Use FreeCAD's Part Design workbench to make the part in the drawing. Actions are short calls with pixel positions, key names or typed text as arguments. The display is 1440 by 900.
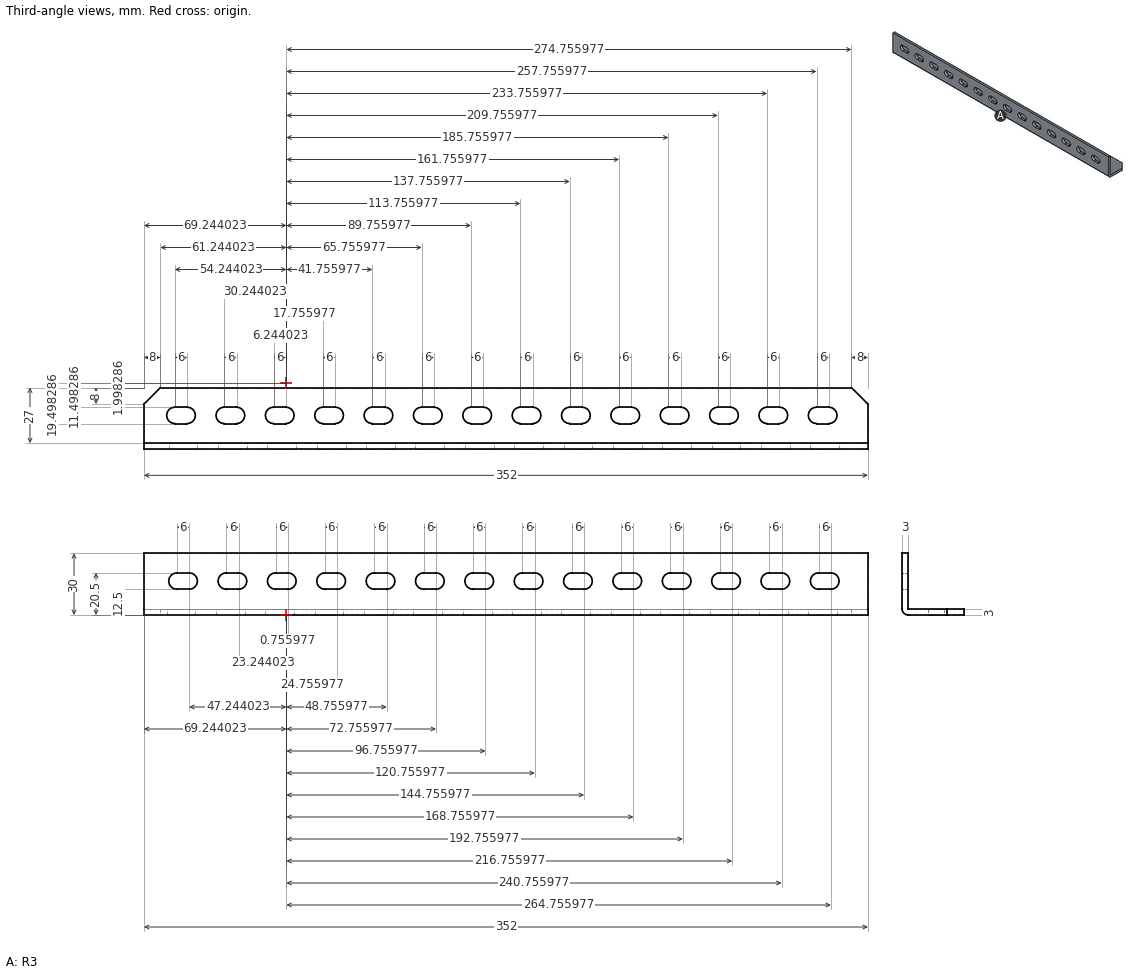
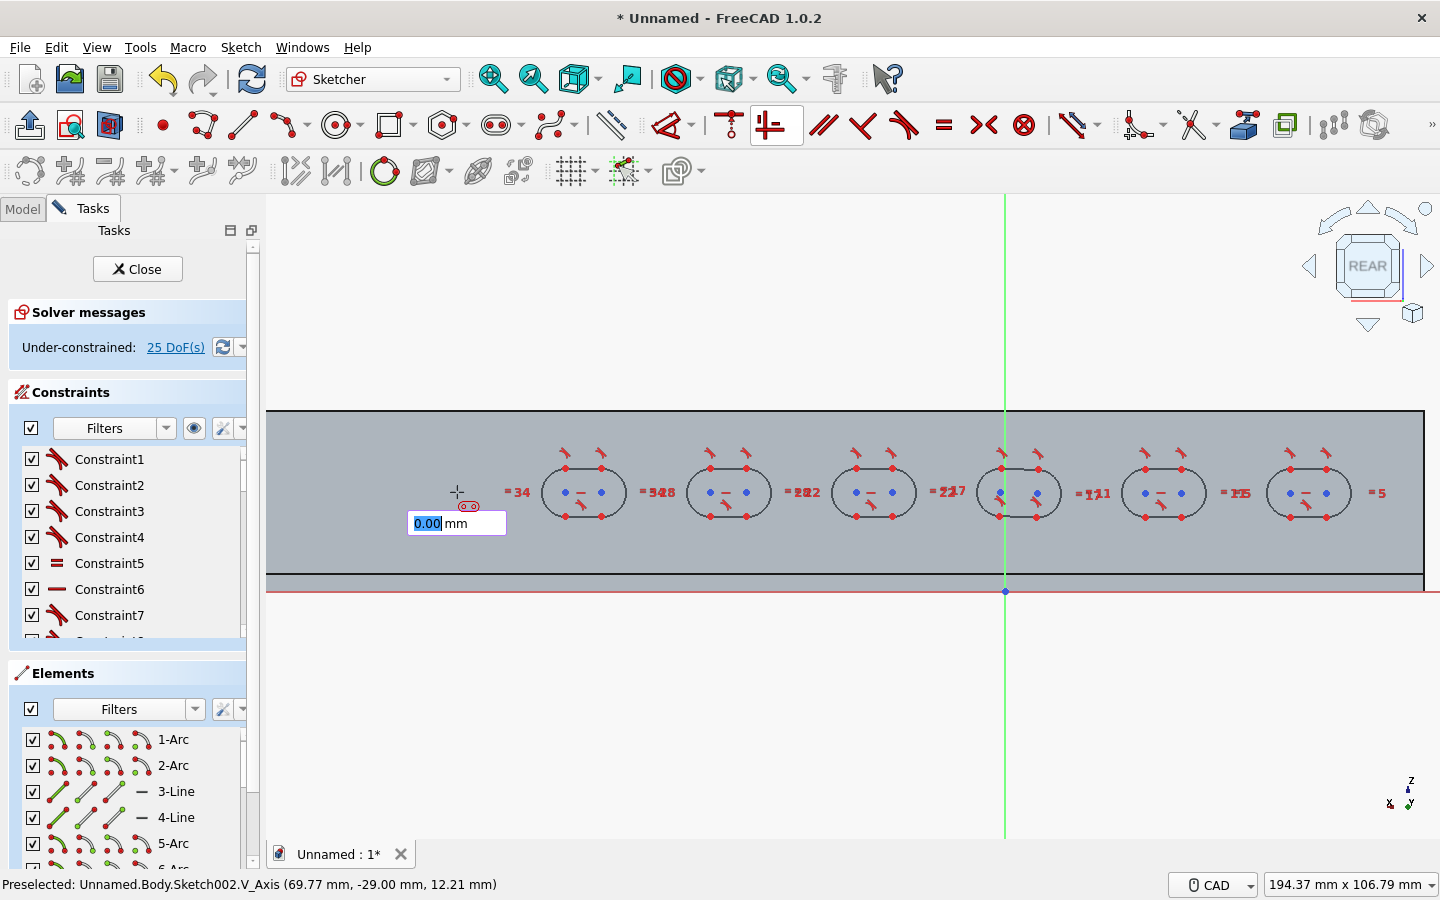
click(439, 516)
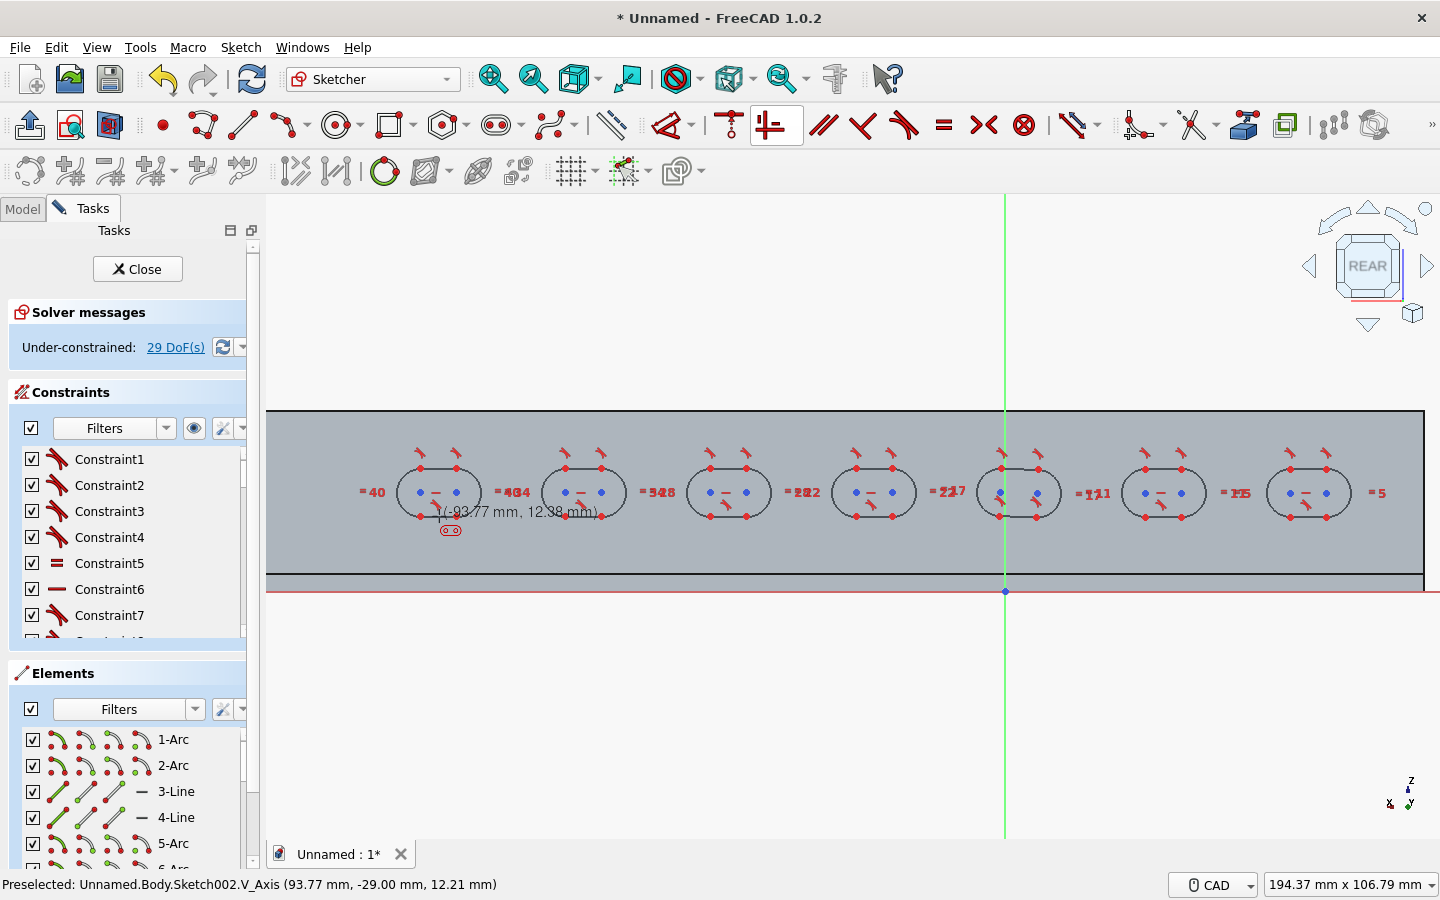
scroll(1028, 509, down, 5)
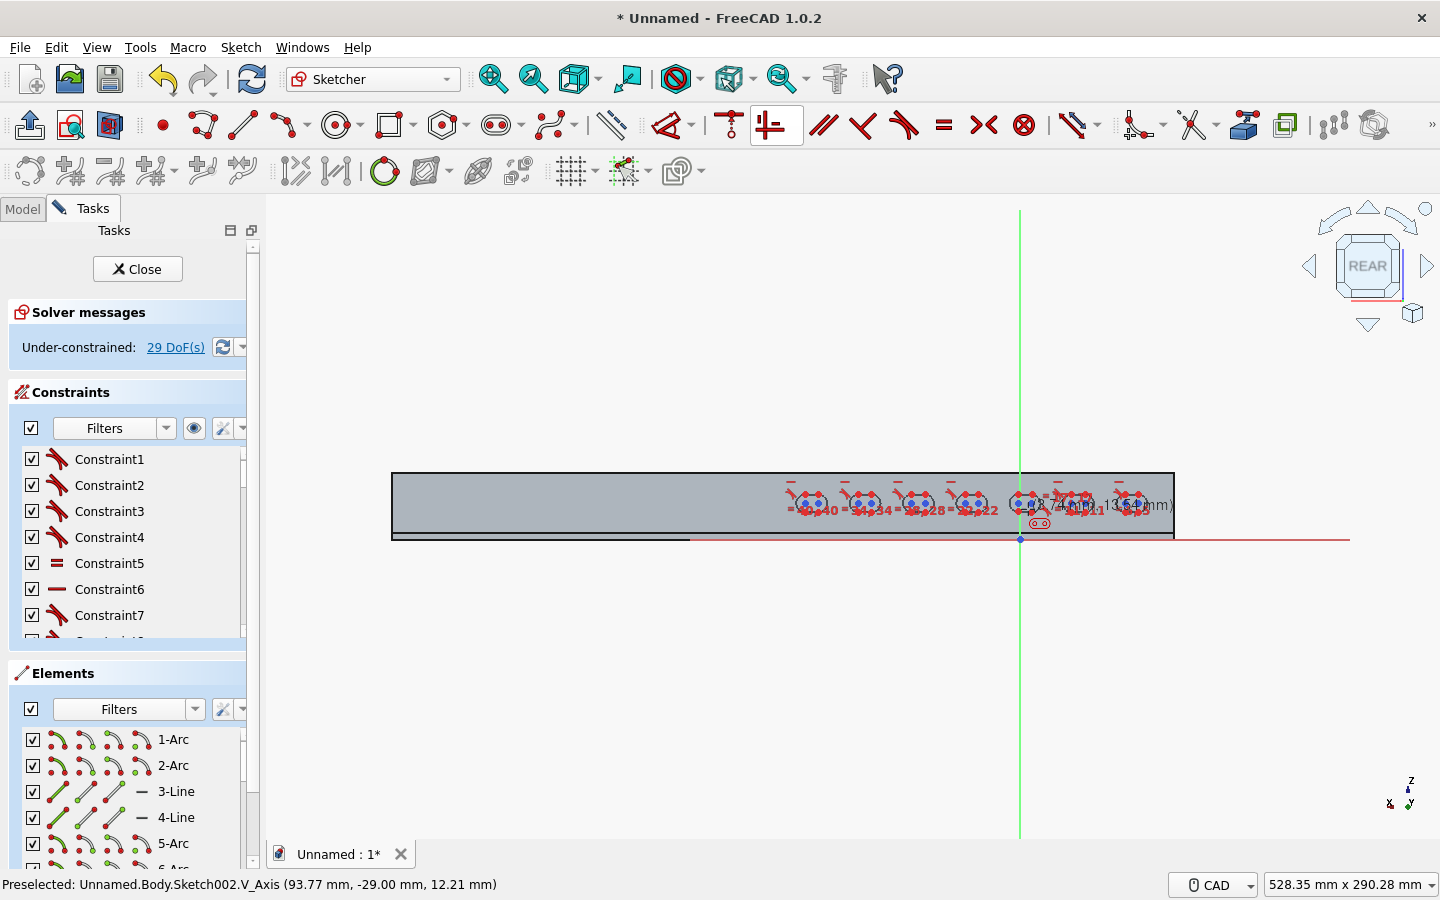
scroll(752, 503, up, 5)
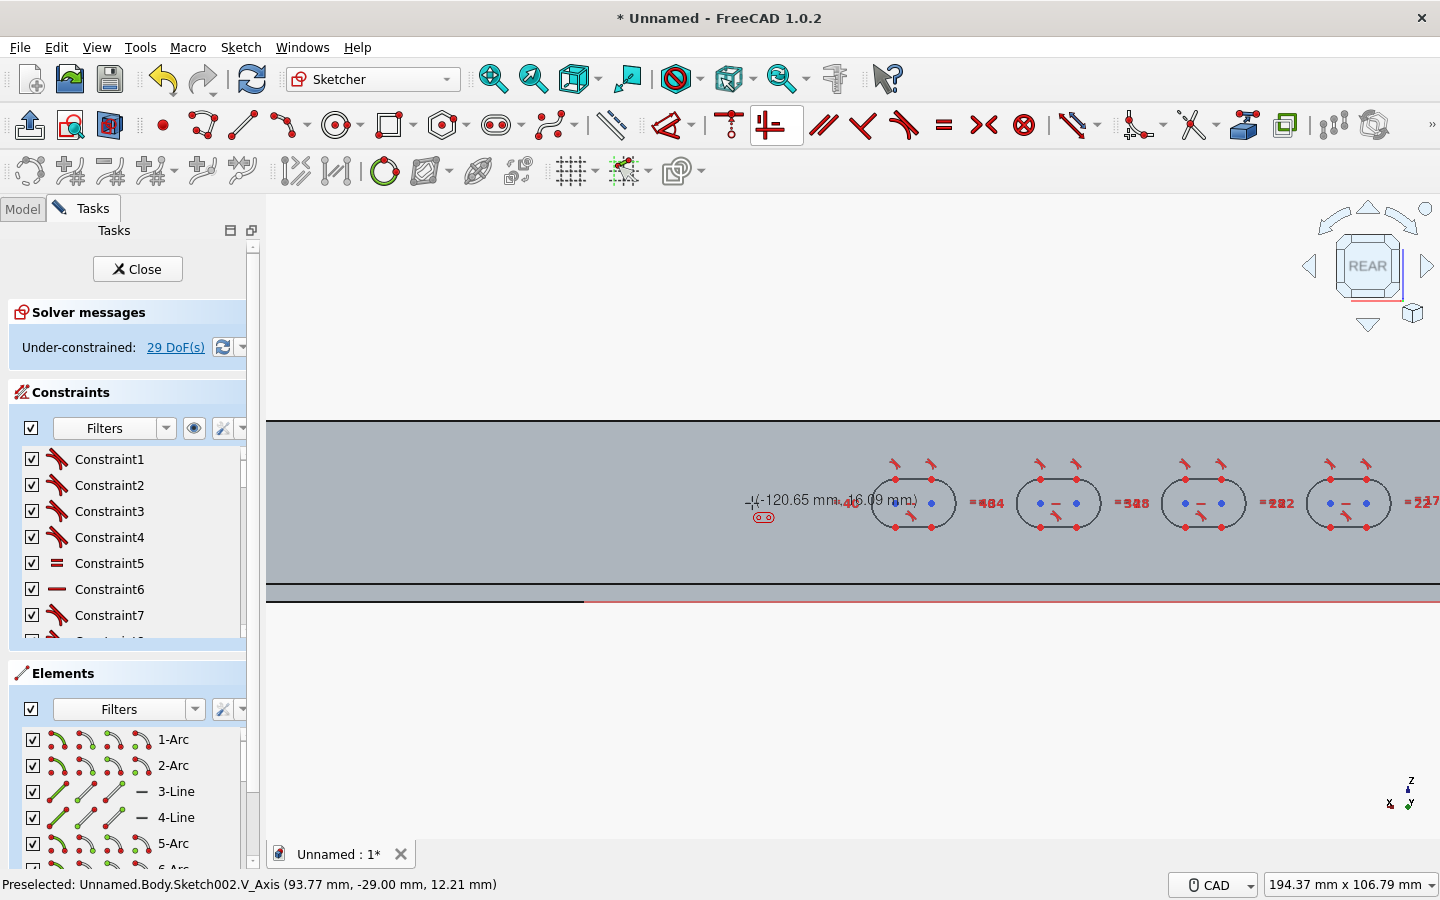
click(751, 502)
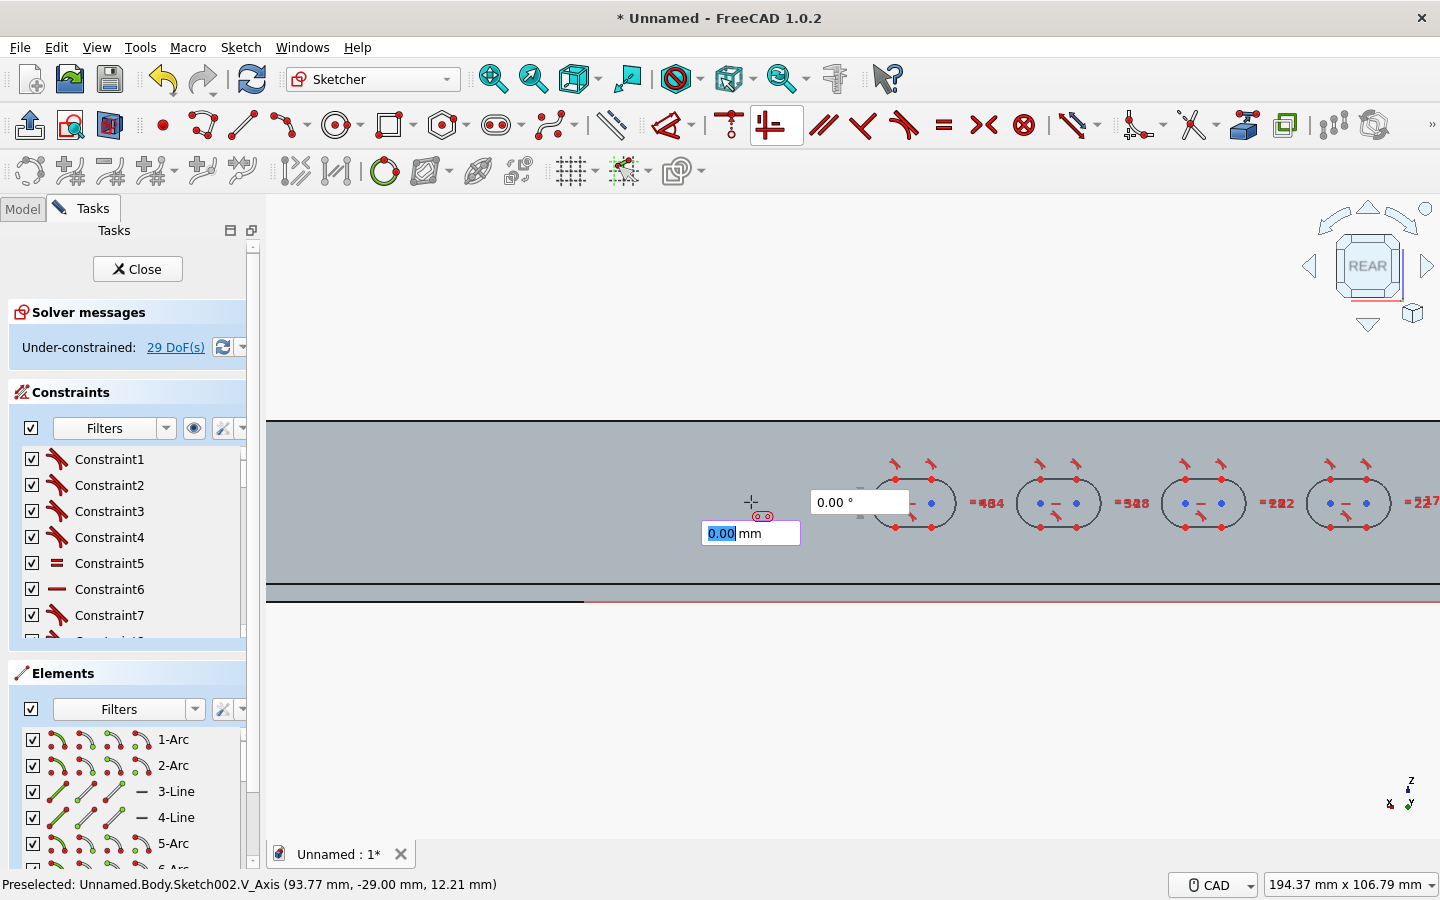
click(787, 502)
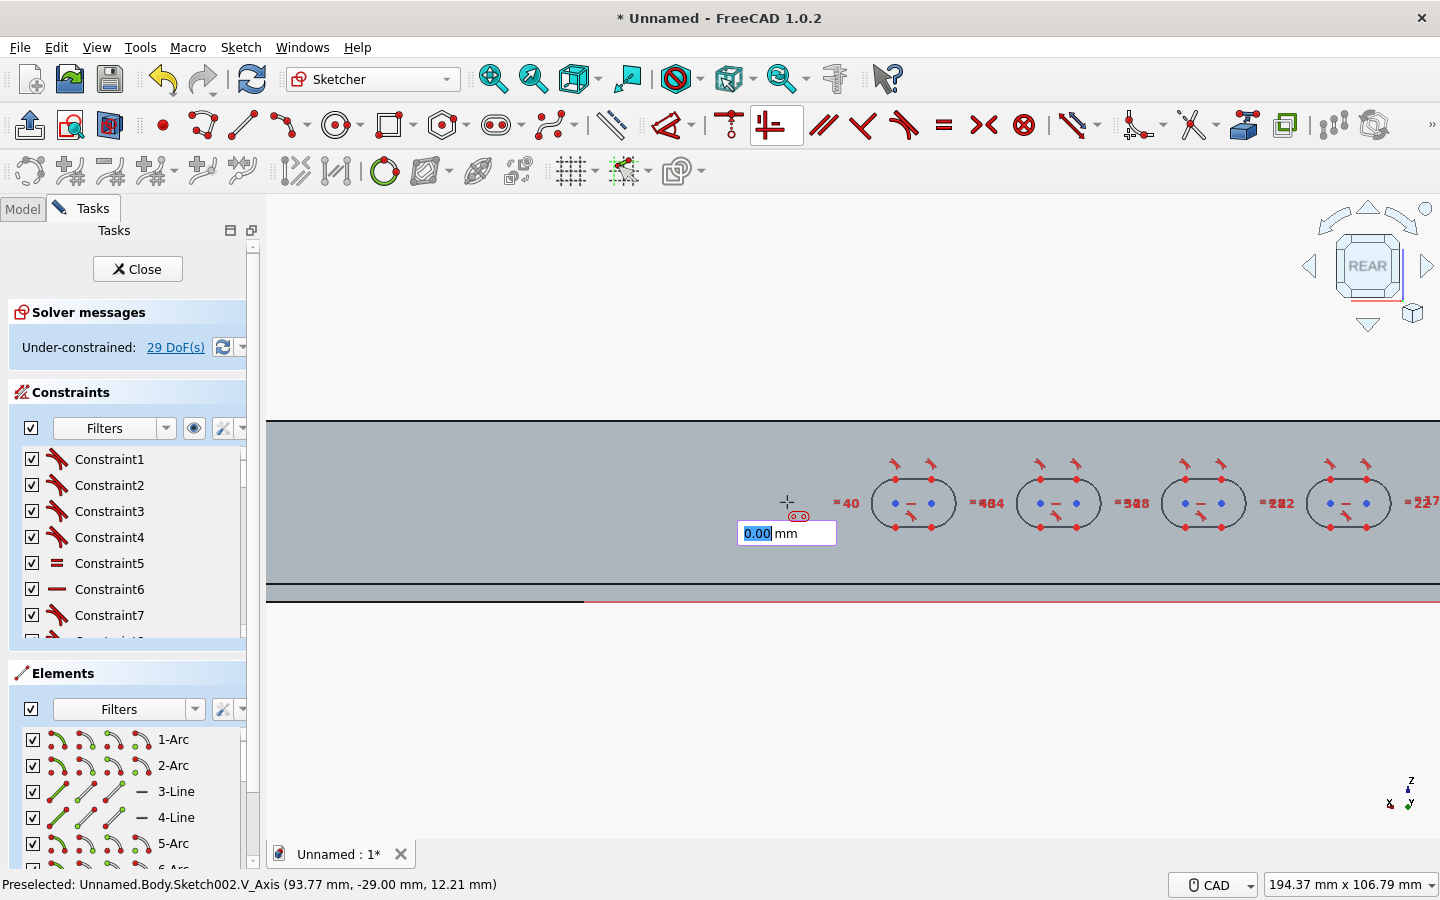
click(769, 527)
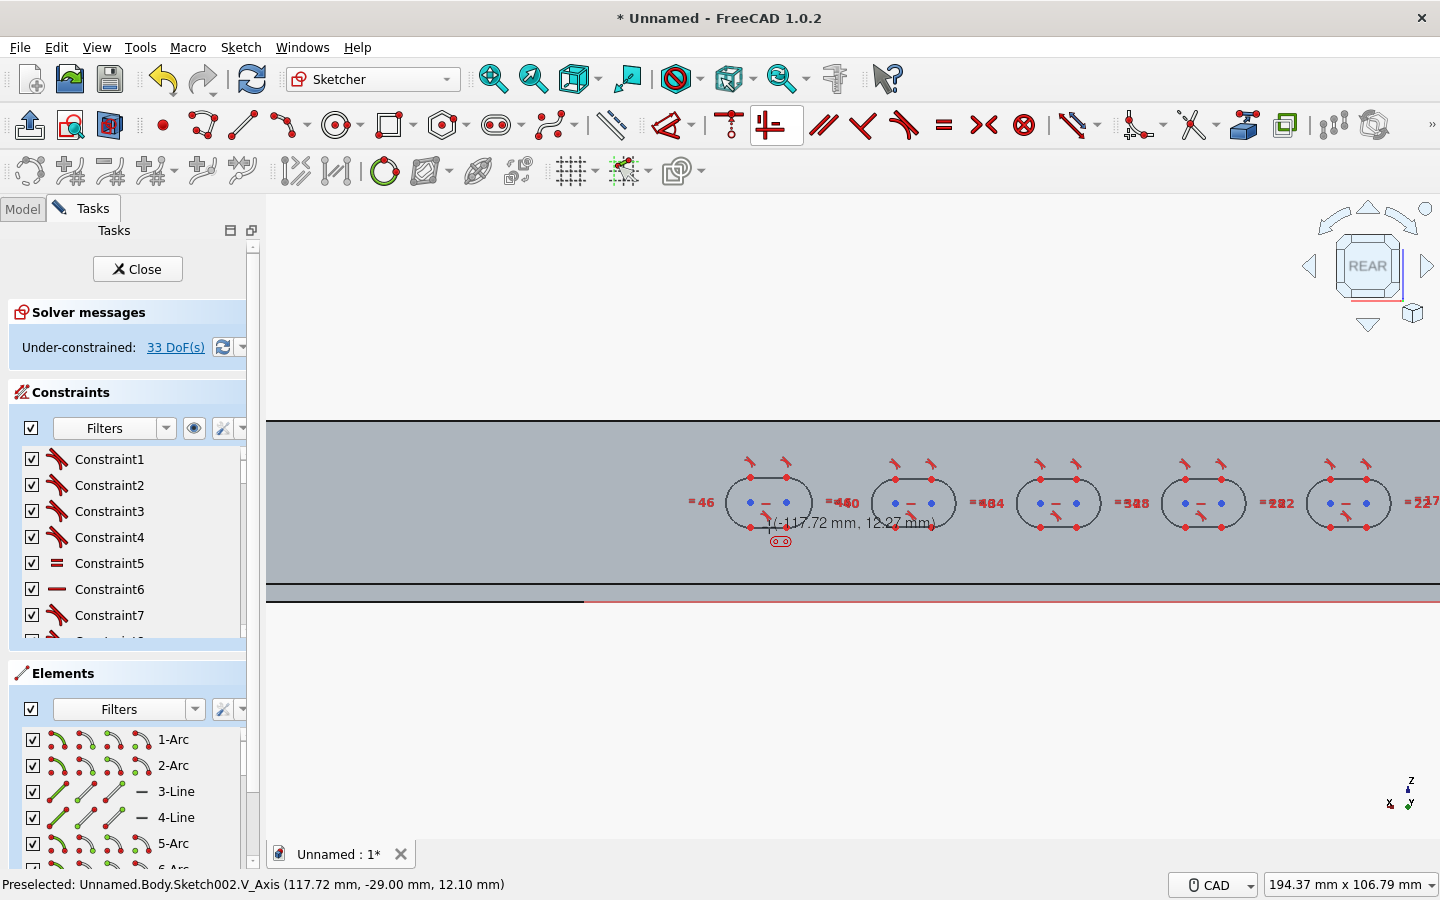
click(606, 502)